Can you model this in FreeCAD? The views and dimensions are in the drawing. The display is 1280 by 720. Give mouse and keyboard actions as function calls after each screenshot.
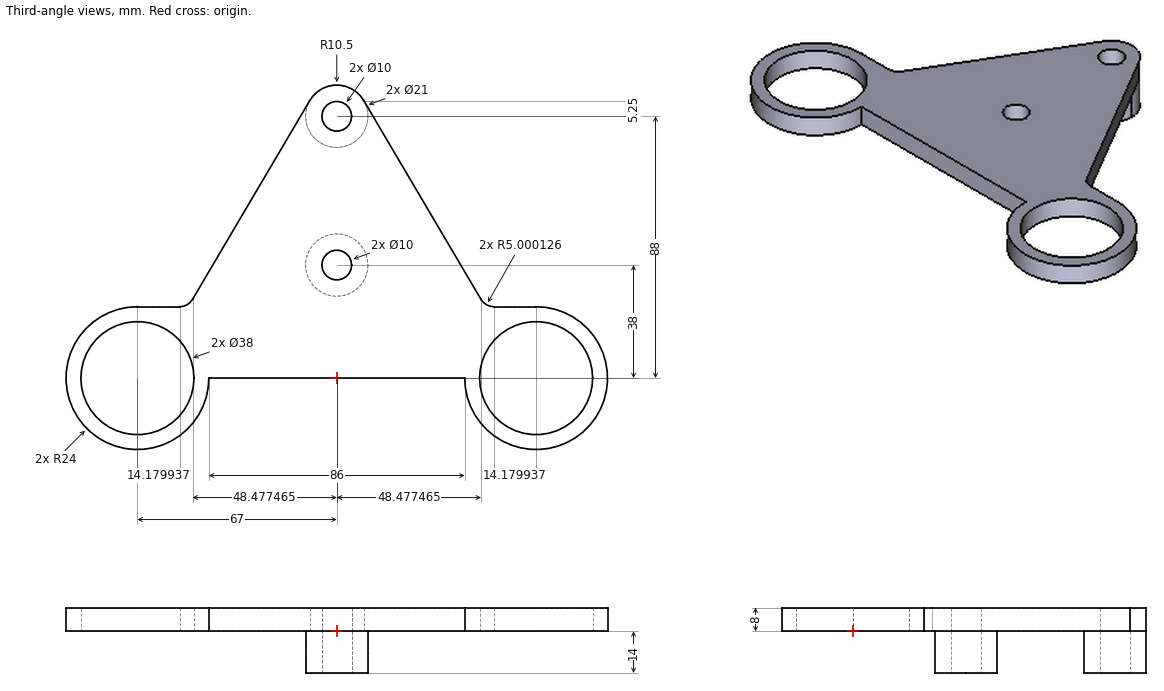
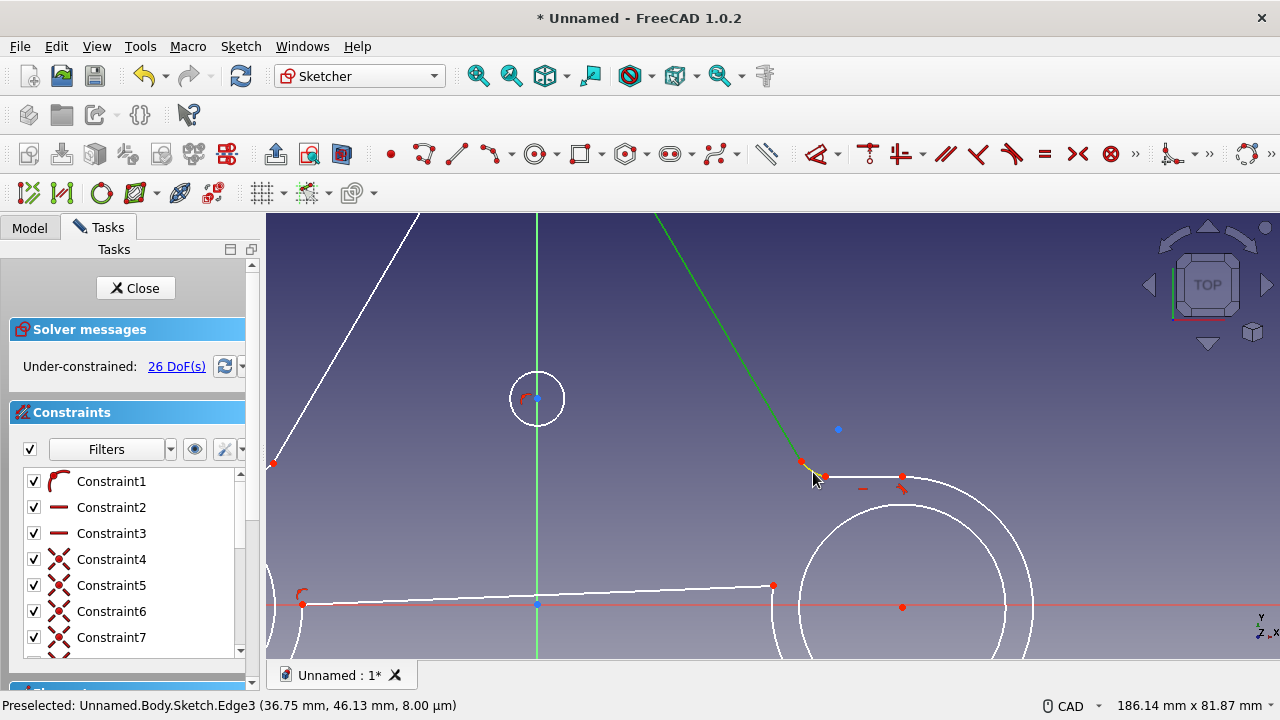
click(812, 471)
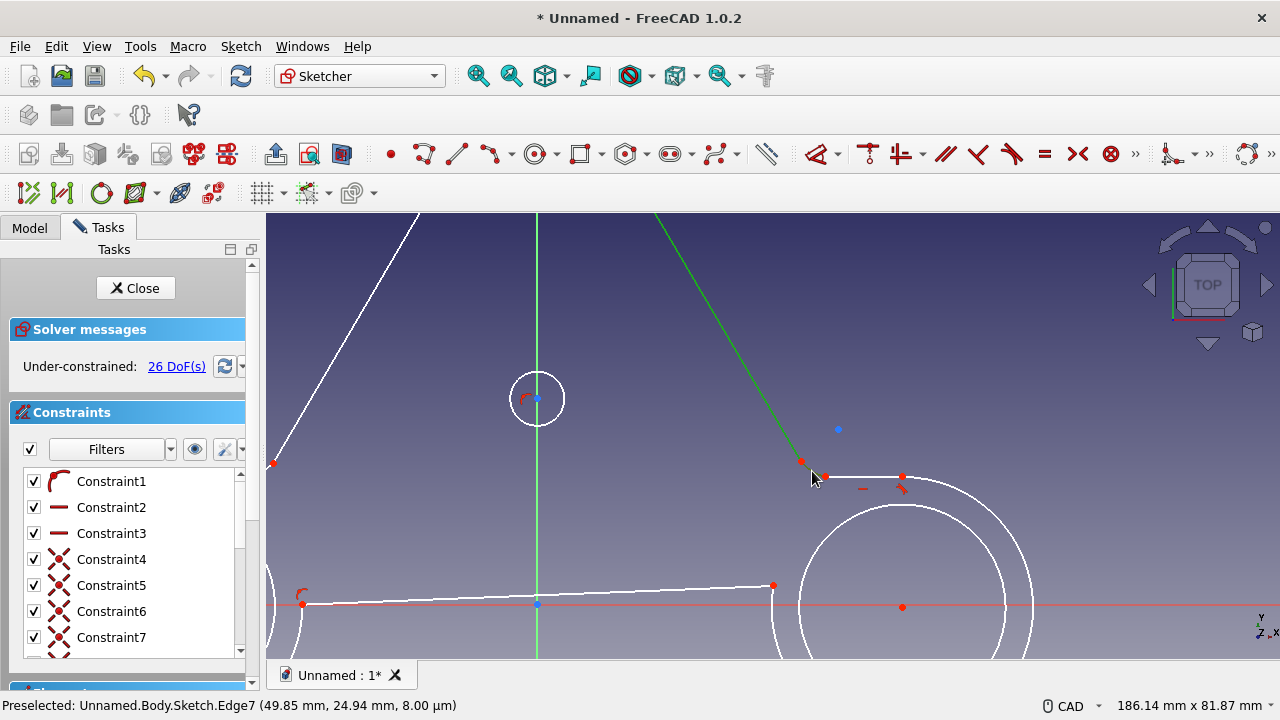
key(t)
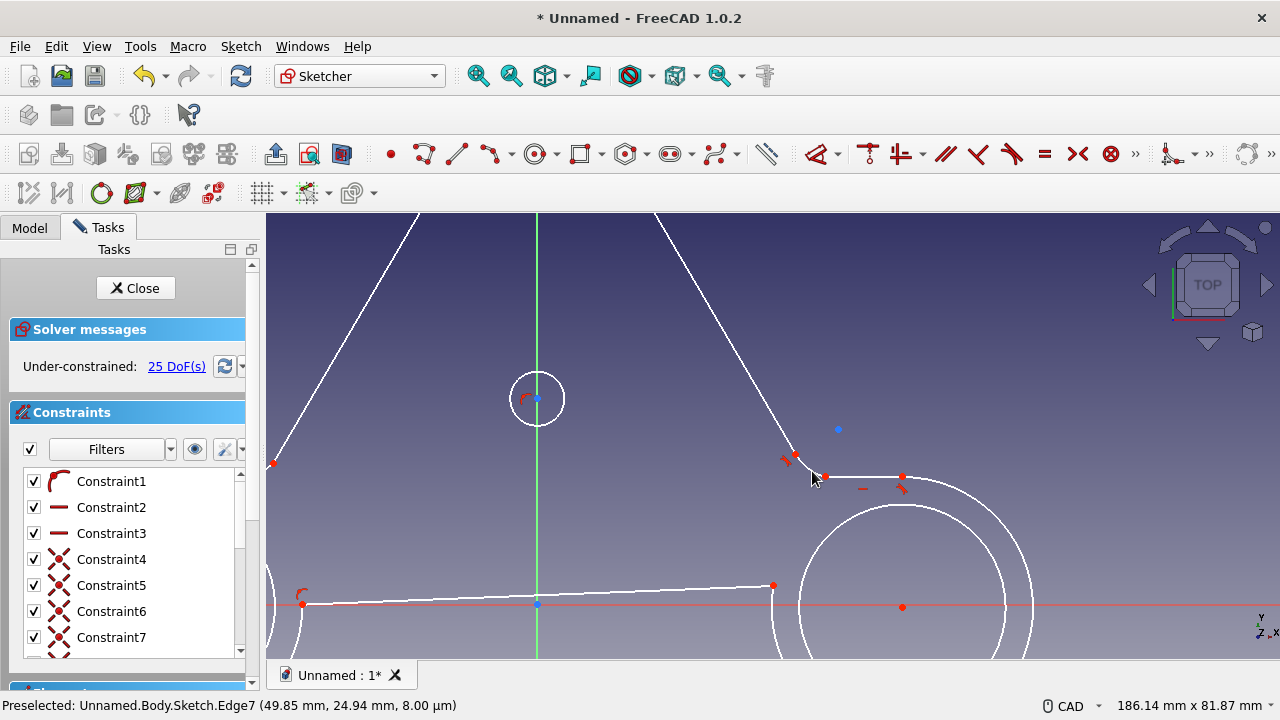
click(337, 354)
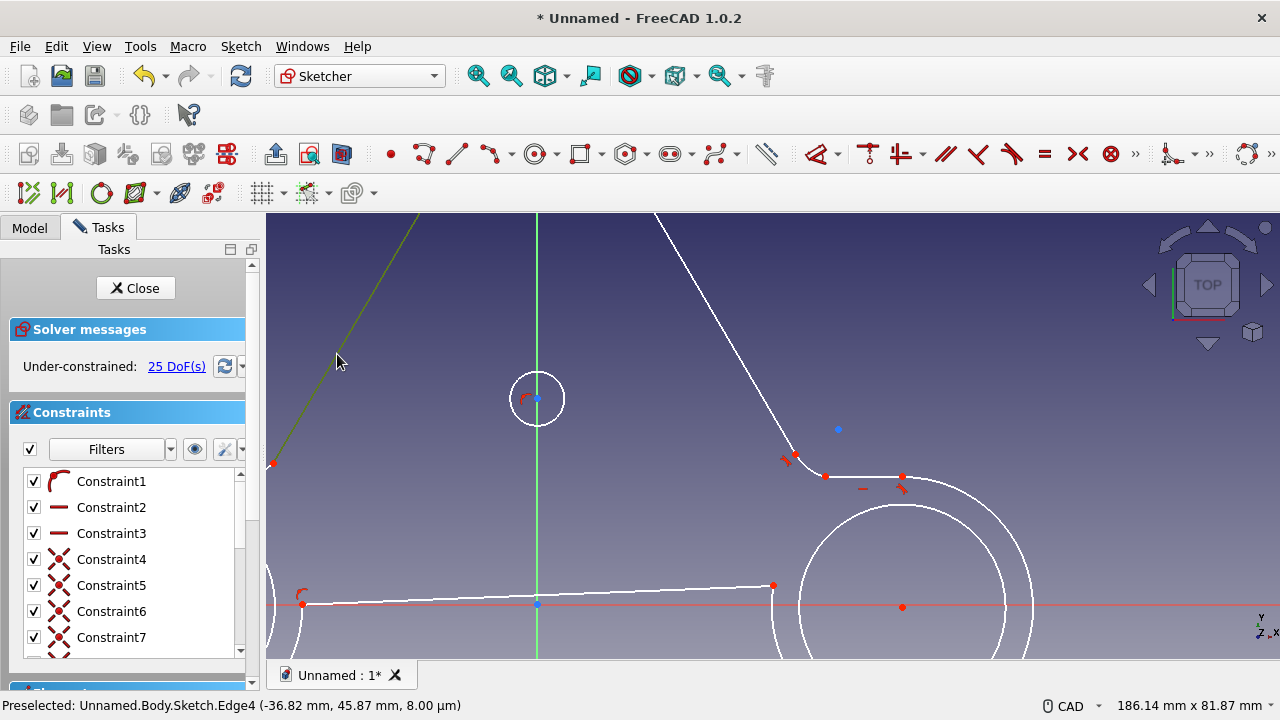
scroll(841, 475, down, 4)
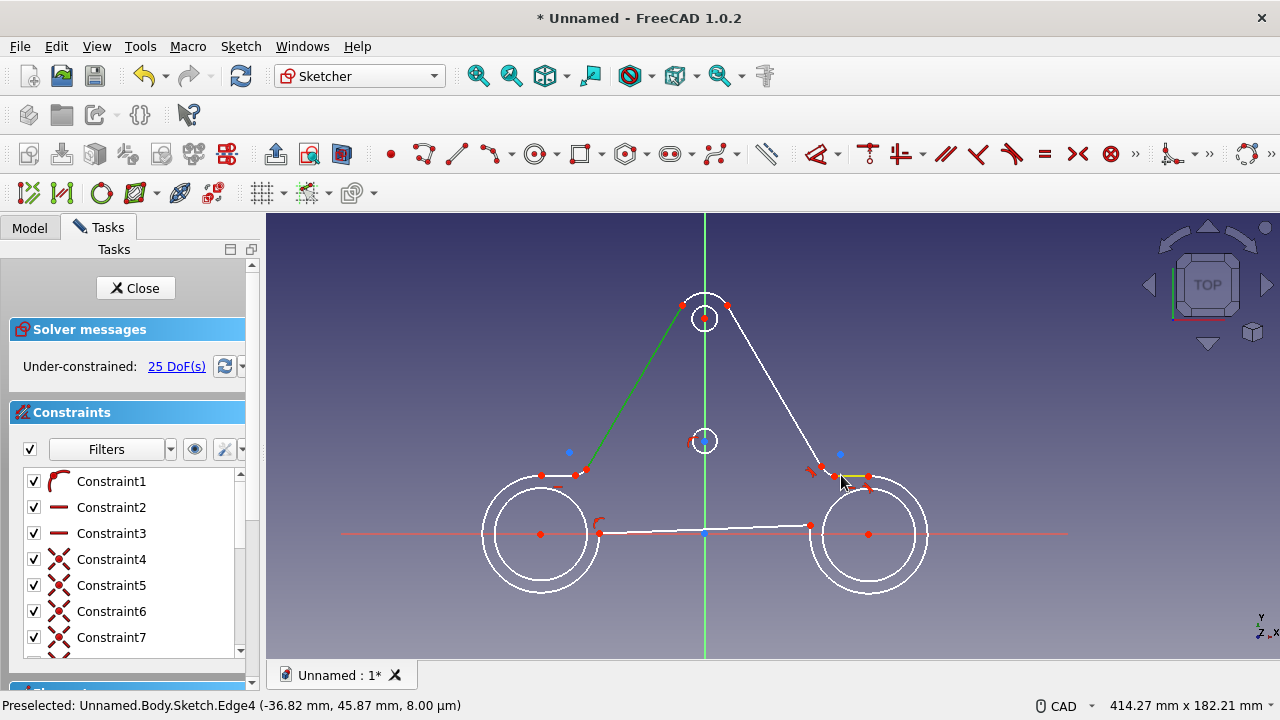
scroll(581, 474, up, 4)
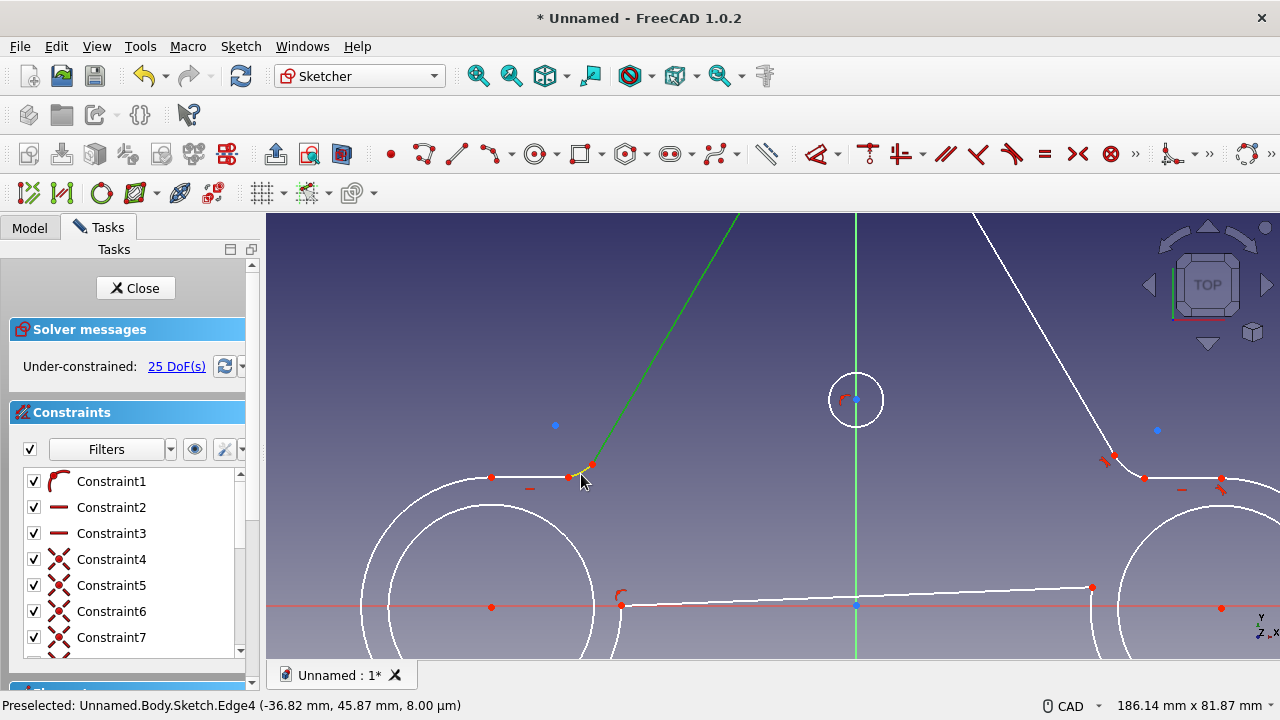
click(581, 472)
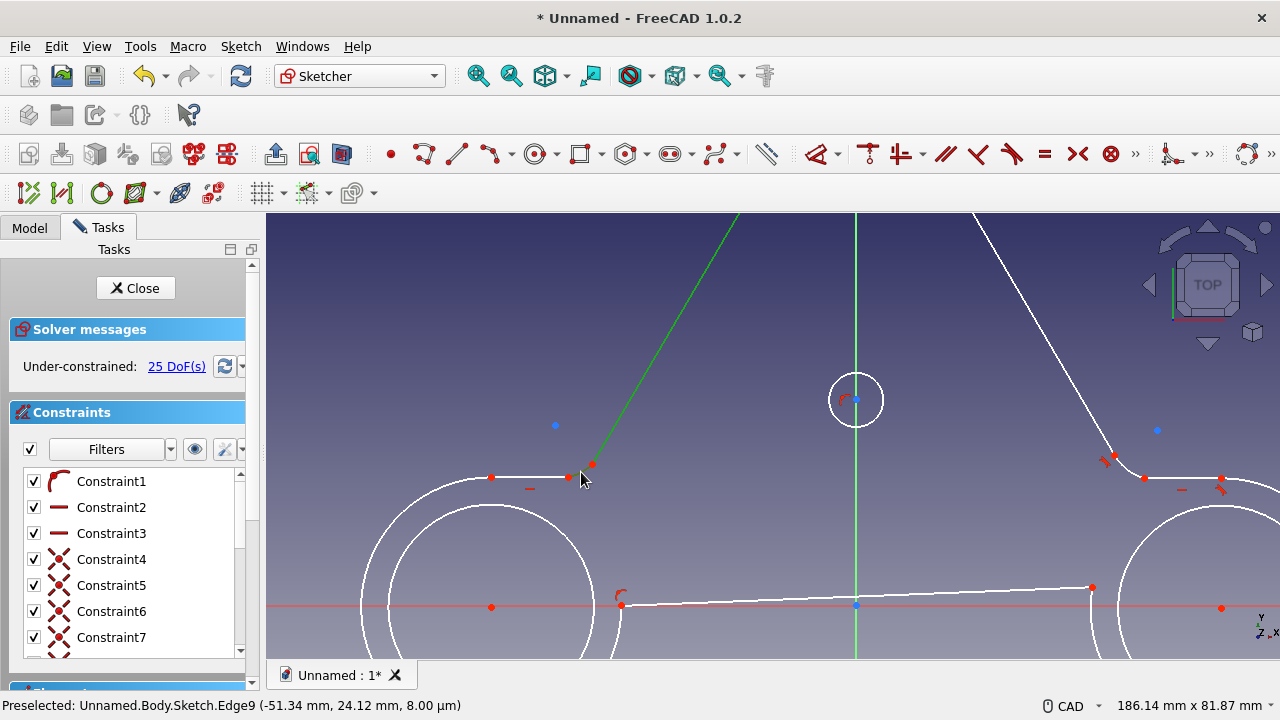
key(t)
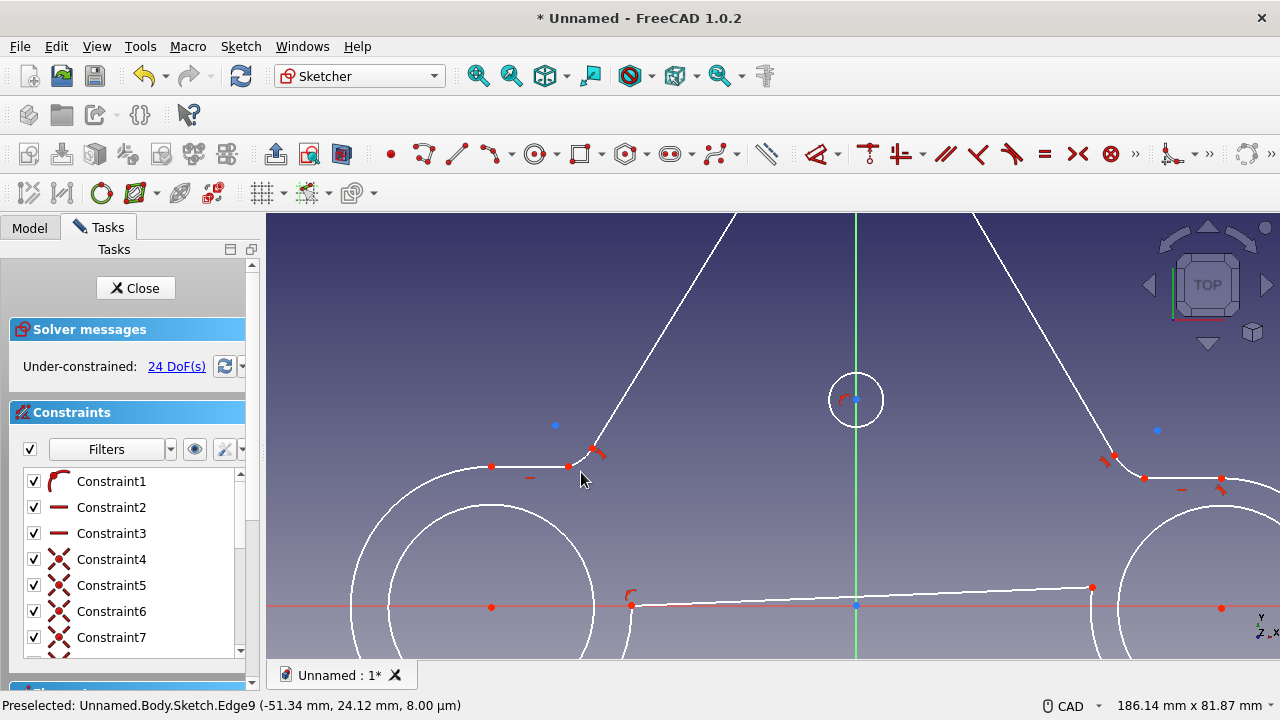
click(545, 467)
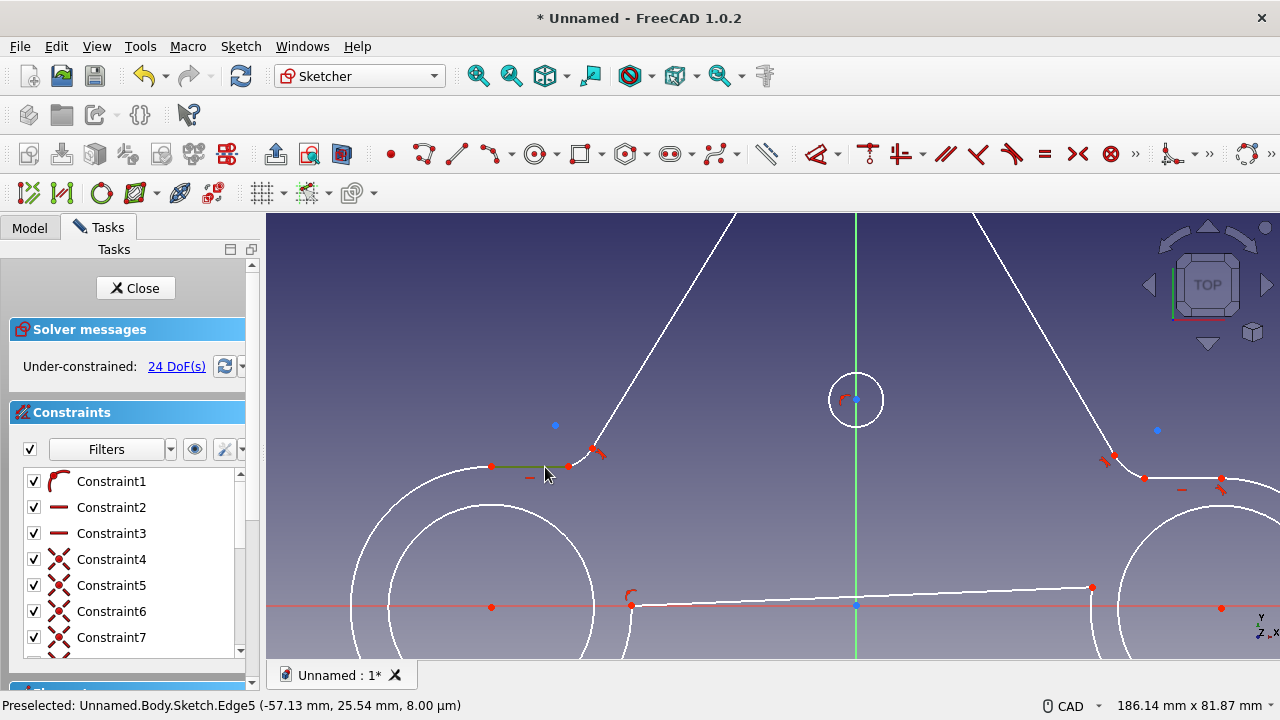
click(352, 585)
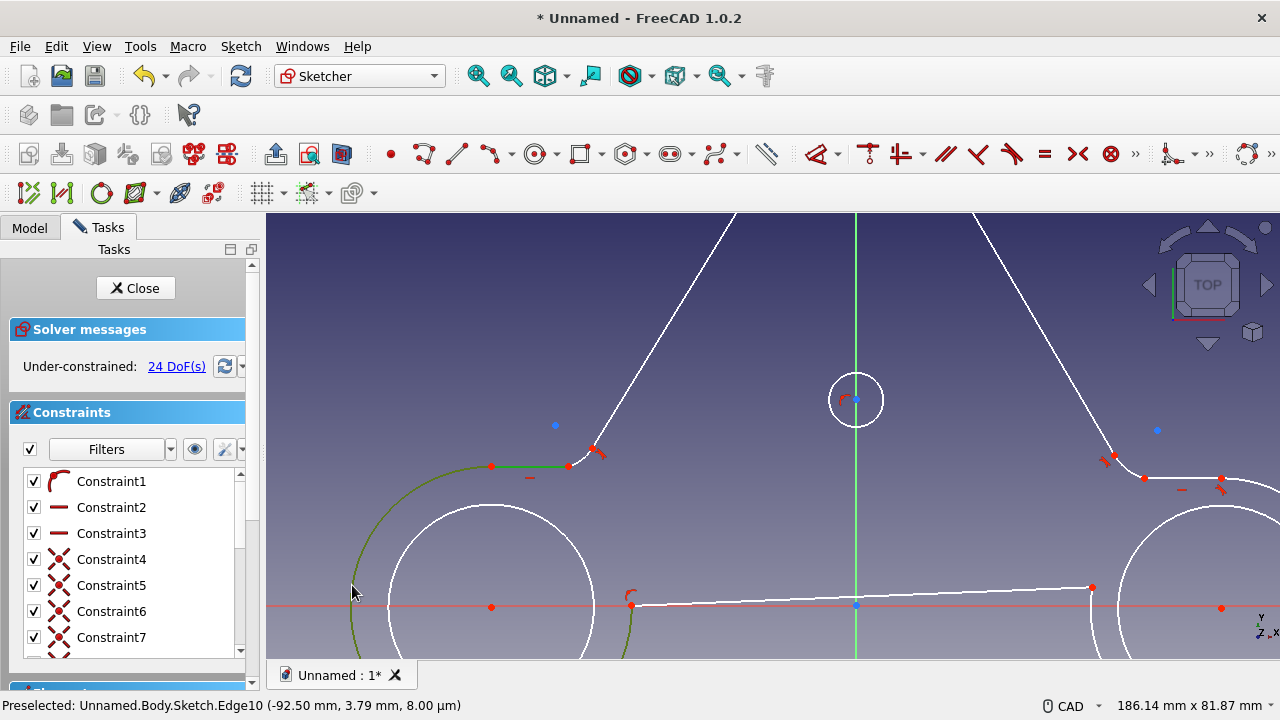
click(1012, 154)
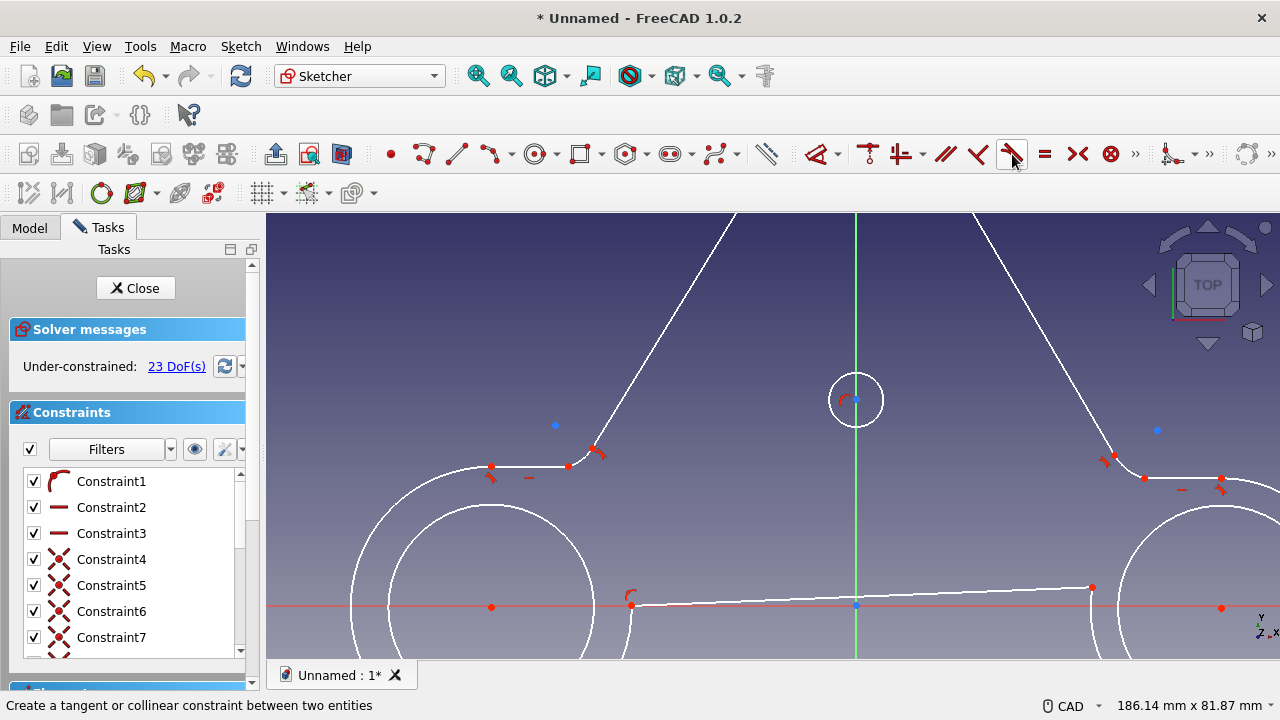
click(954, 593)